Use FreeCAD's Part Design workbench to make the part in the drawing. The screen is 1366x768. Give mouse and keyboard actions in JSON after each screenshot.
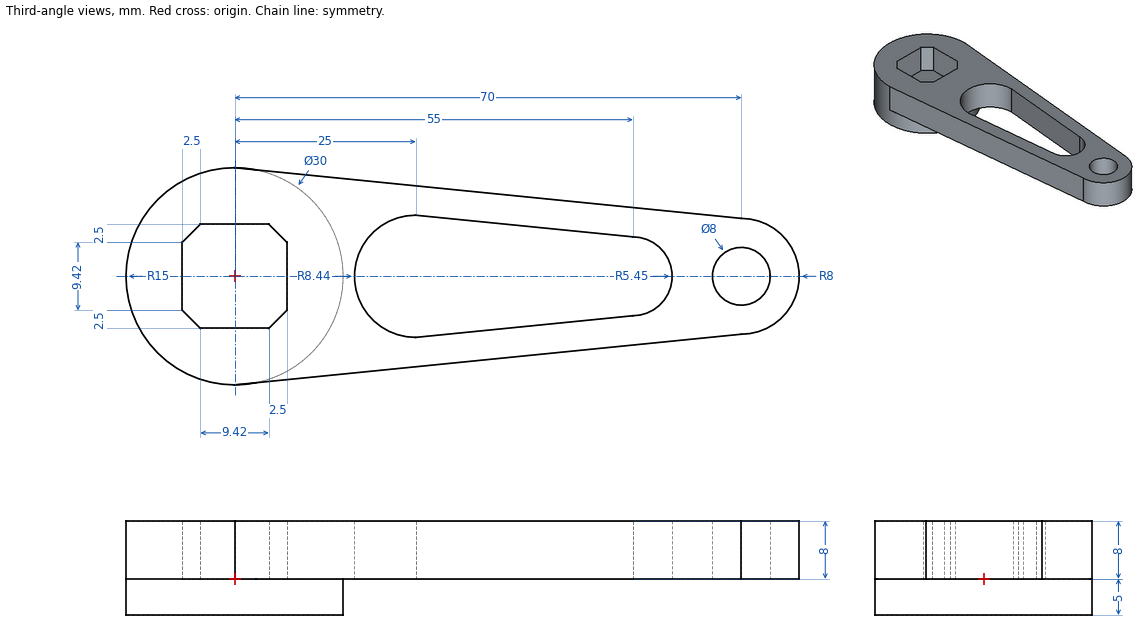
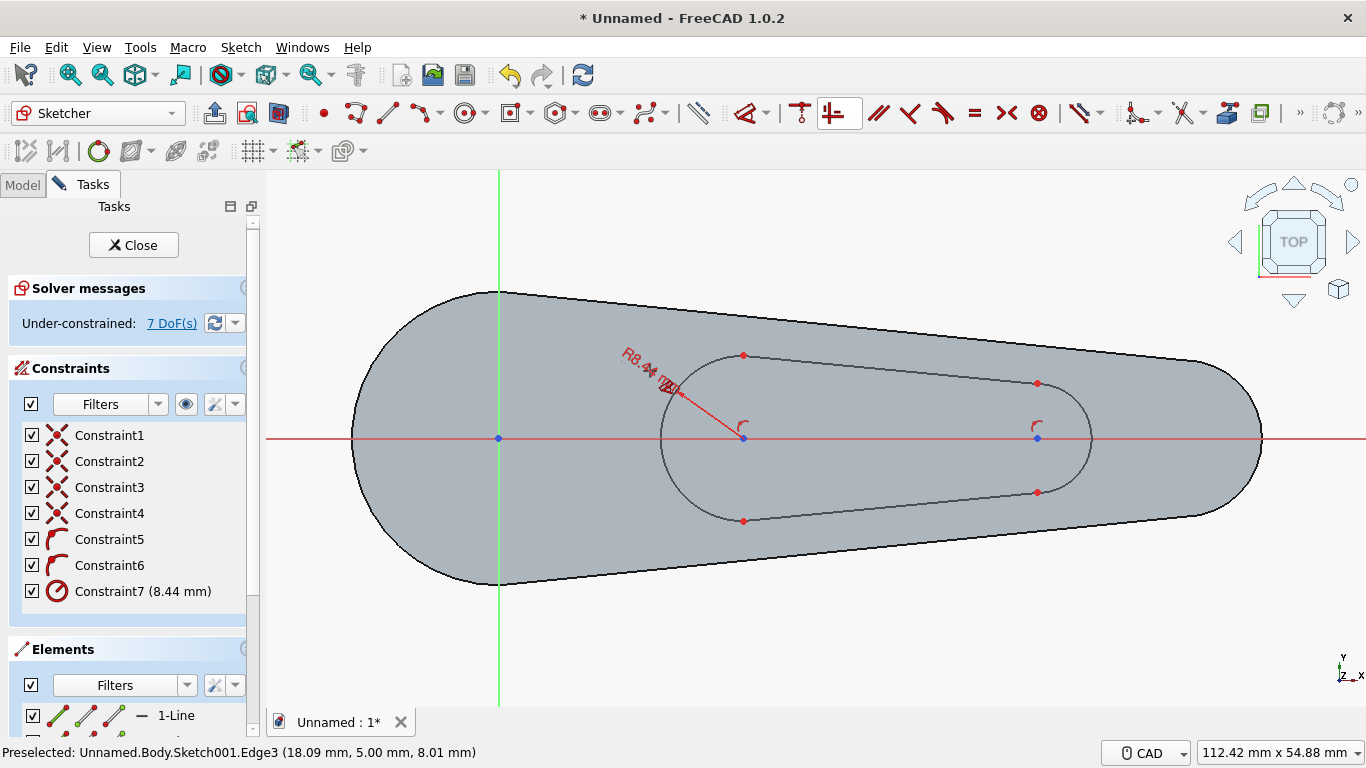
{"action": "left_click", "coordinate": [1081, 471]}
{"action": "left_click", "coordinate": [1107, 490]}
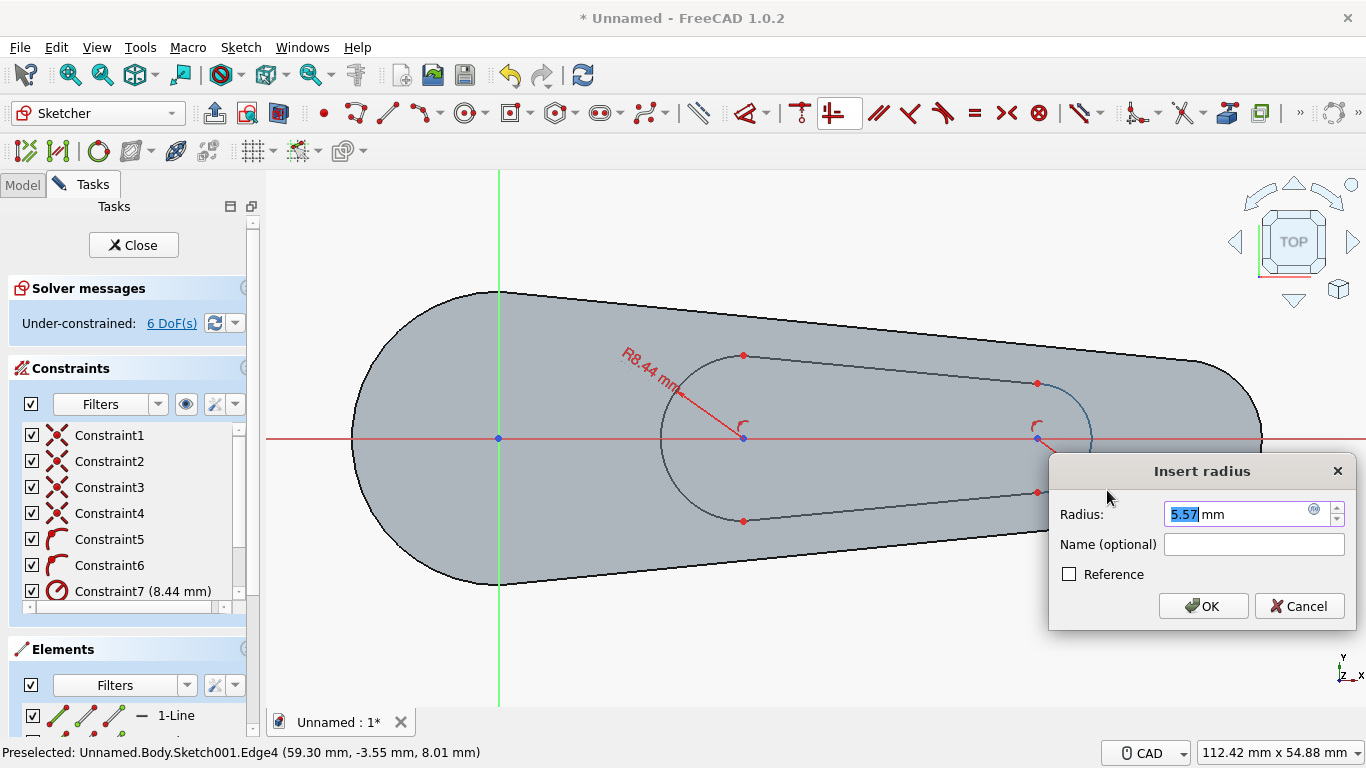
{"action": "type", "text": "5.45"}
{"action": "key", "text": "Return"}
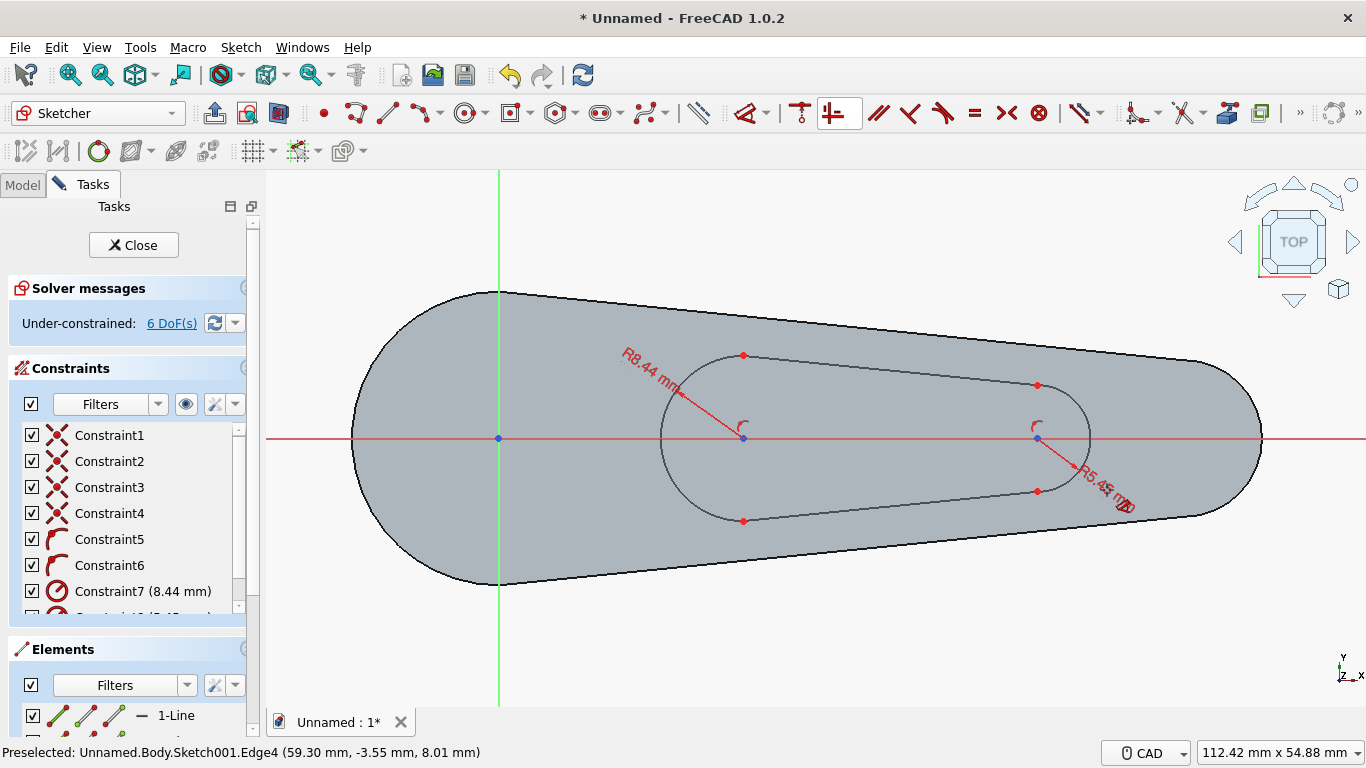
{"action": "left_click", "coordinate": [1037, 385]}
{"action": "left_click", "coordinate": [644, 351]}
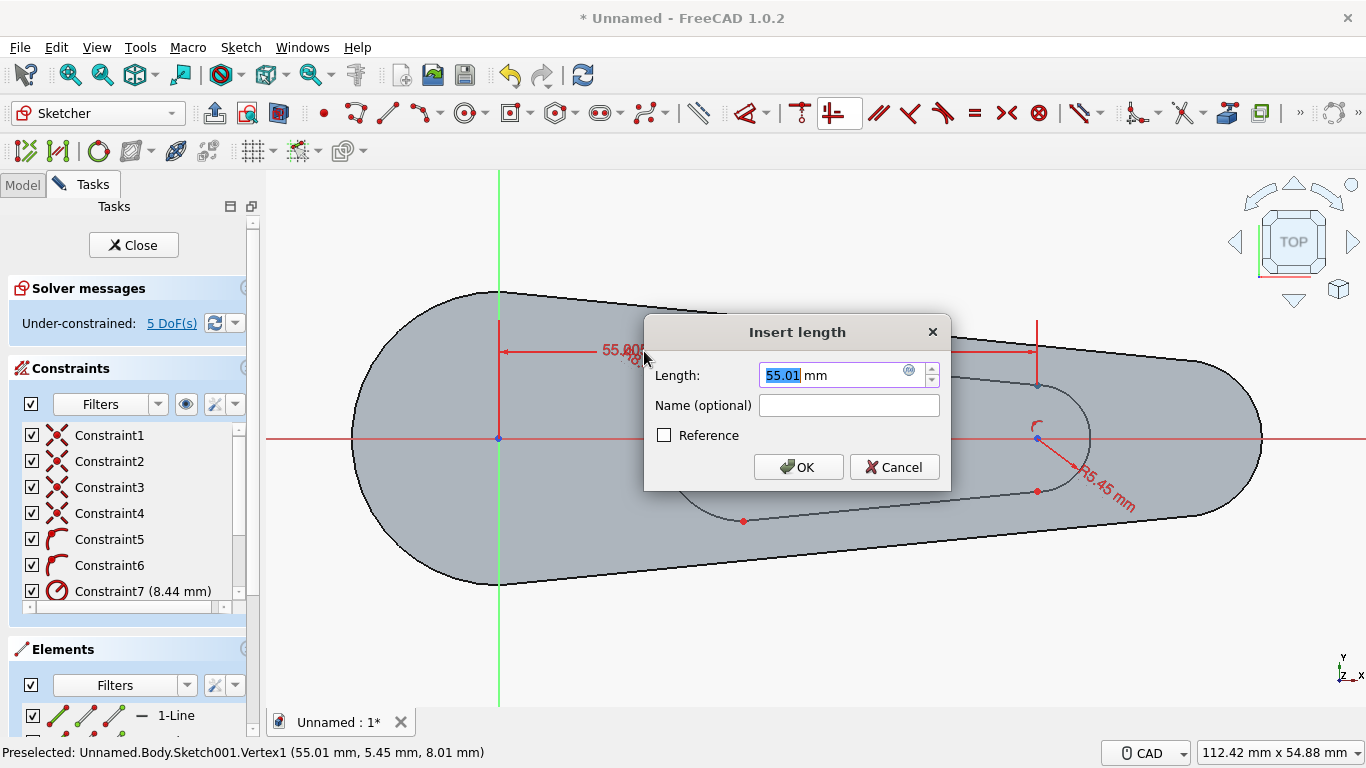
{"action": "type", "text": "55"}
{"action": "key", "text": "Return"}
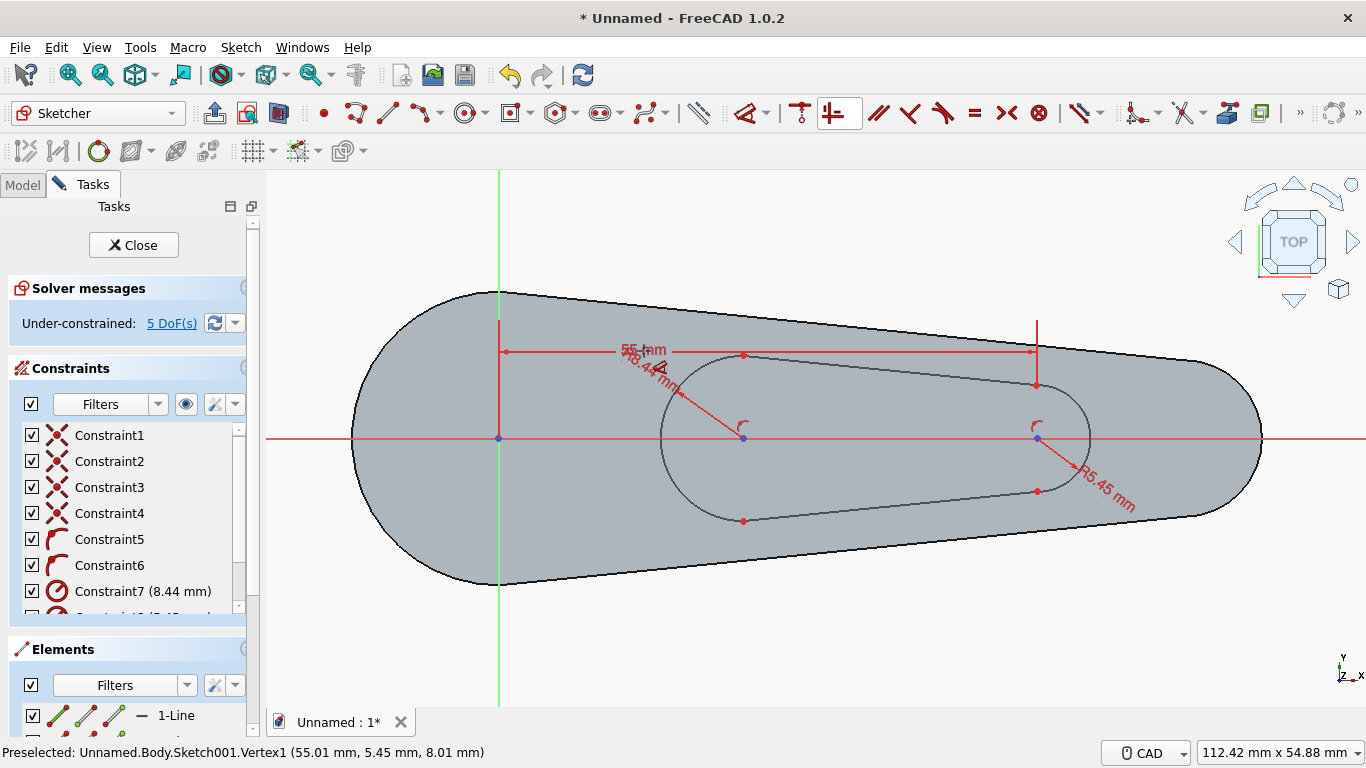
{"action": "left_click", "coordinate": [743, 356]}
{"action": "left_click", "coordinate": [621, 322]}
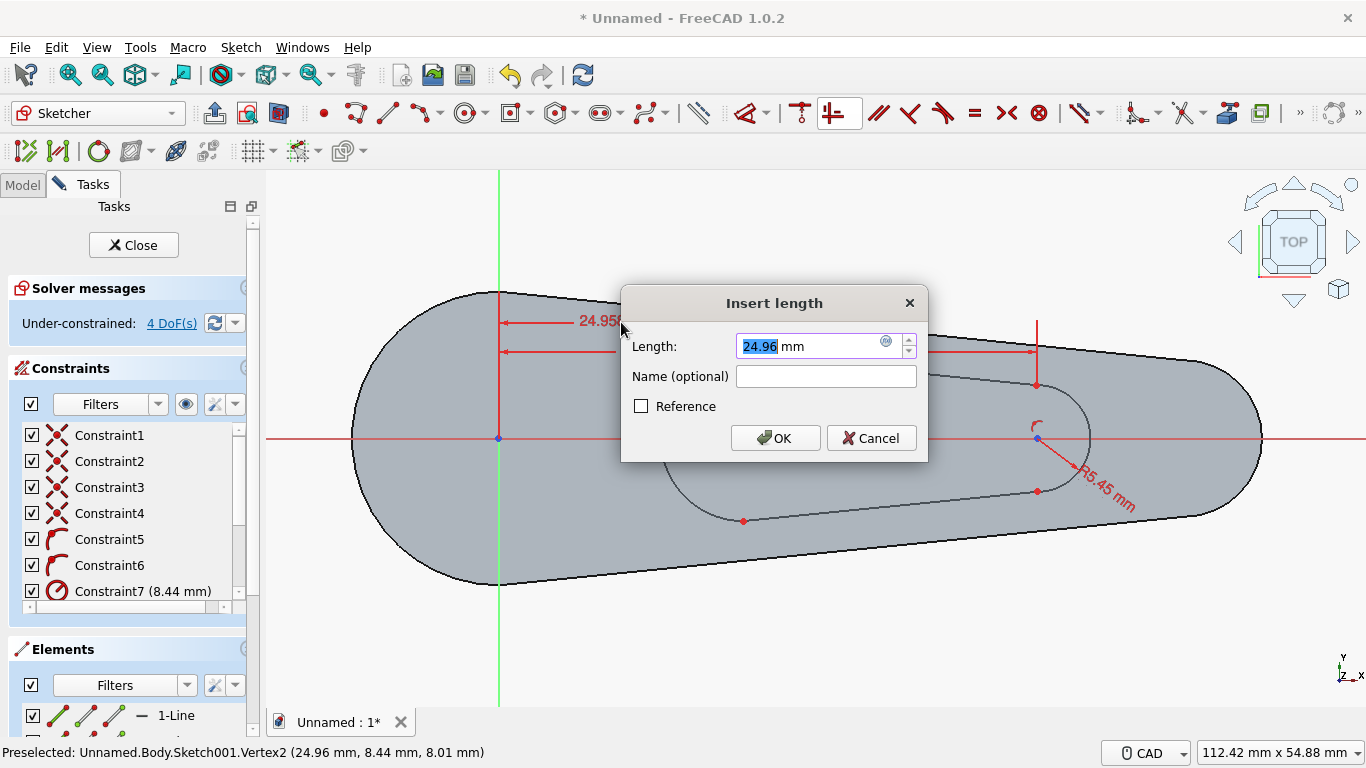
{"action": "type", "text": "25"}
{"action": "key", "text": "Return"}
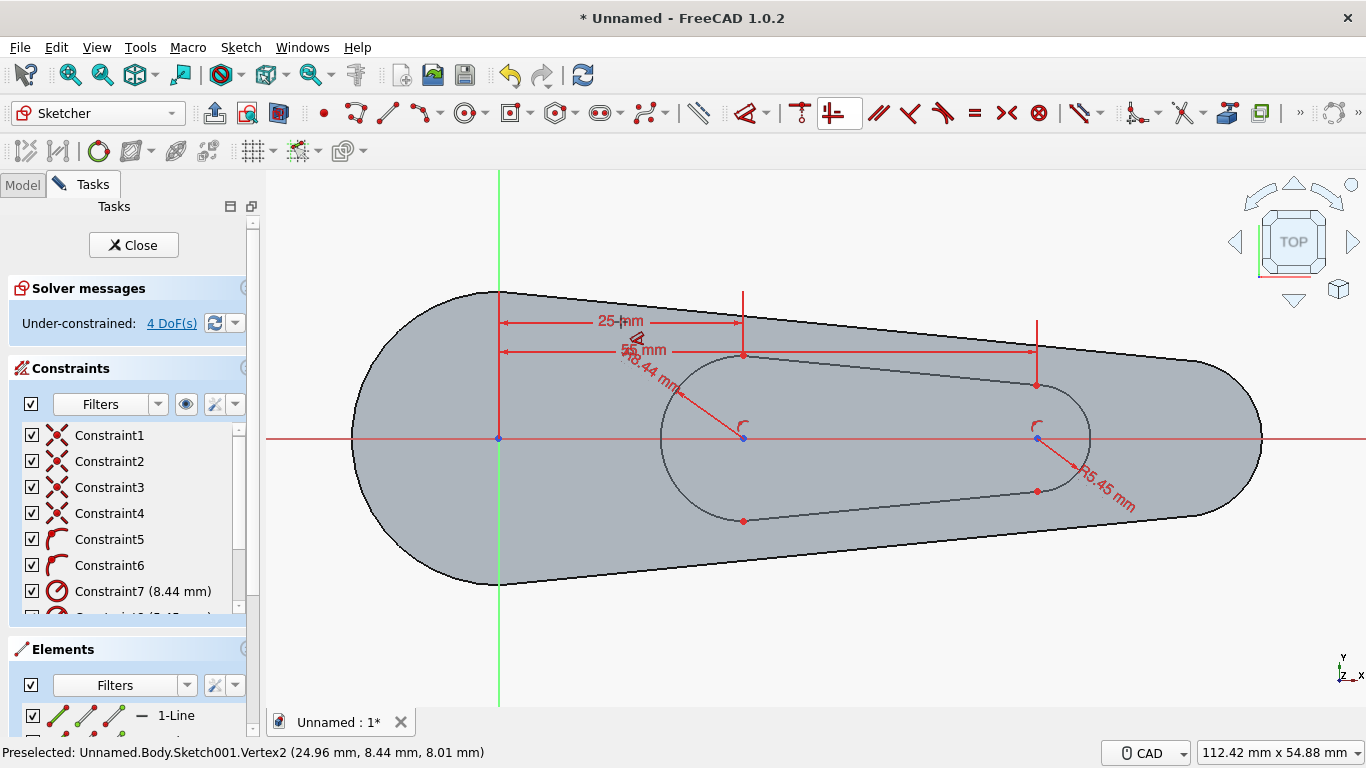
{"action": "left_click", "coordinate": [743, 521]}
{"action": "left_click", "coordinate": [621, 555]}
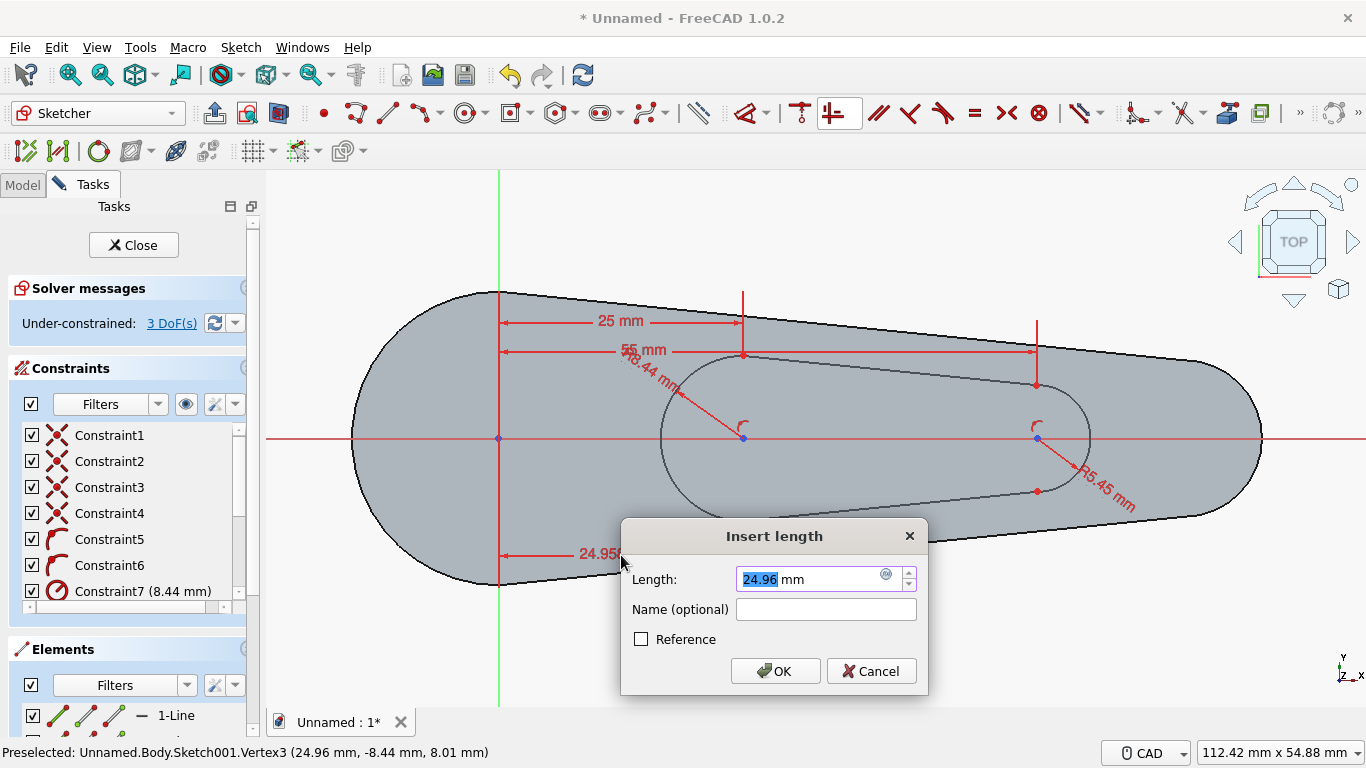
{"action": "type", "text": "25"}
{"action": "key", "text": "Return"}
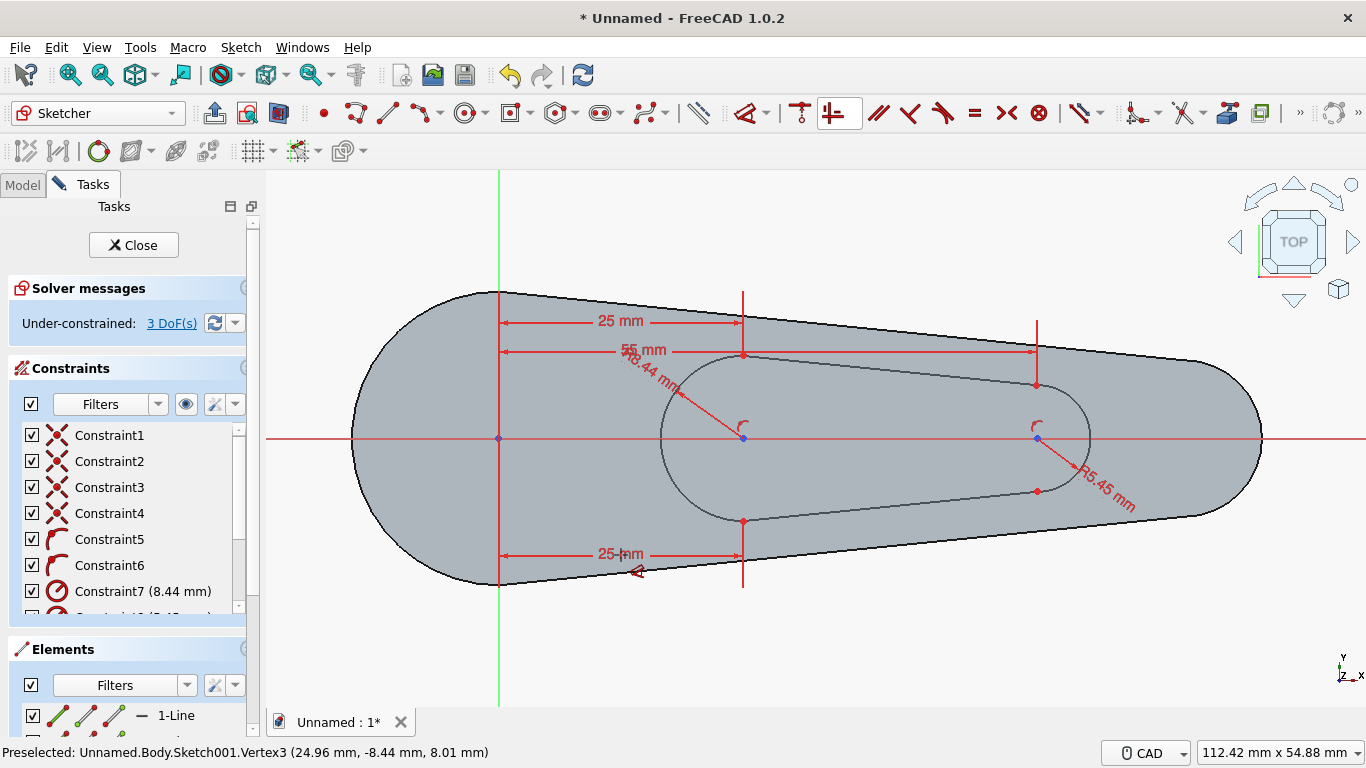
{"action": "left_click", "coordinate": [1037, 492]}
{"action": "left_click", "coordinate": [644, 526]}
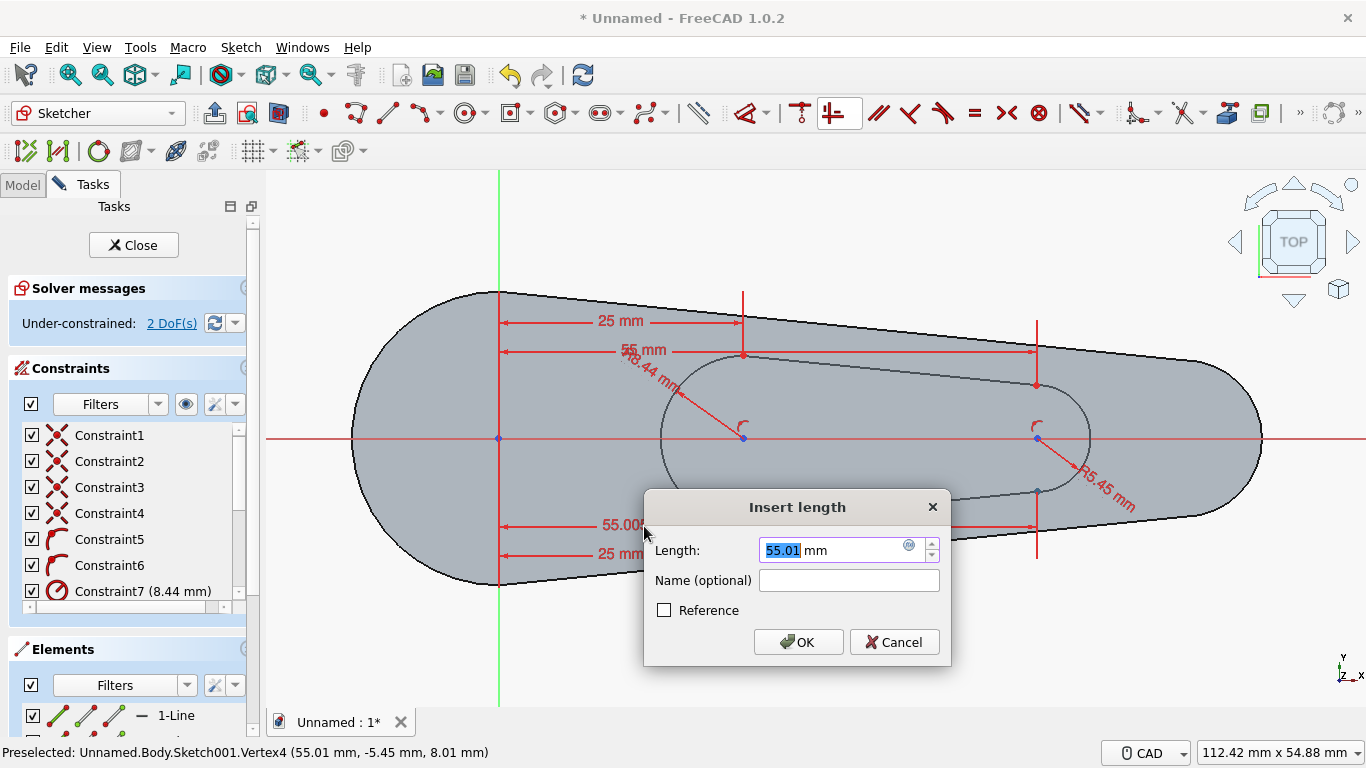
{"action": "type", "text": "55"}
{"action": "key", "text": "Return"}